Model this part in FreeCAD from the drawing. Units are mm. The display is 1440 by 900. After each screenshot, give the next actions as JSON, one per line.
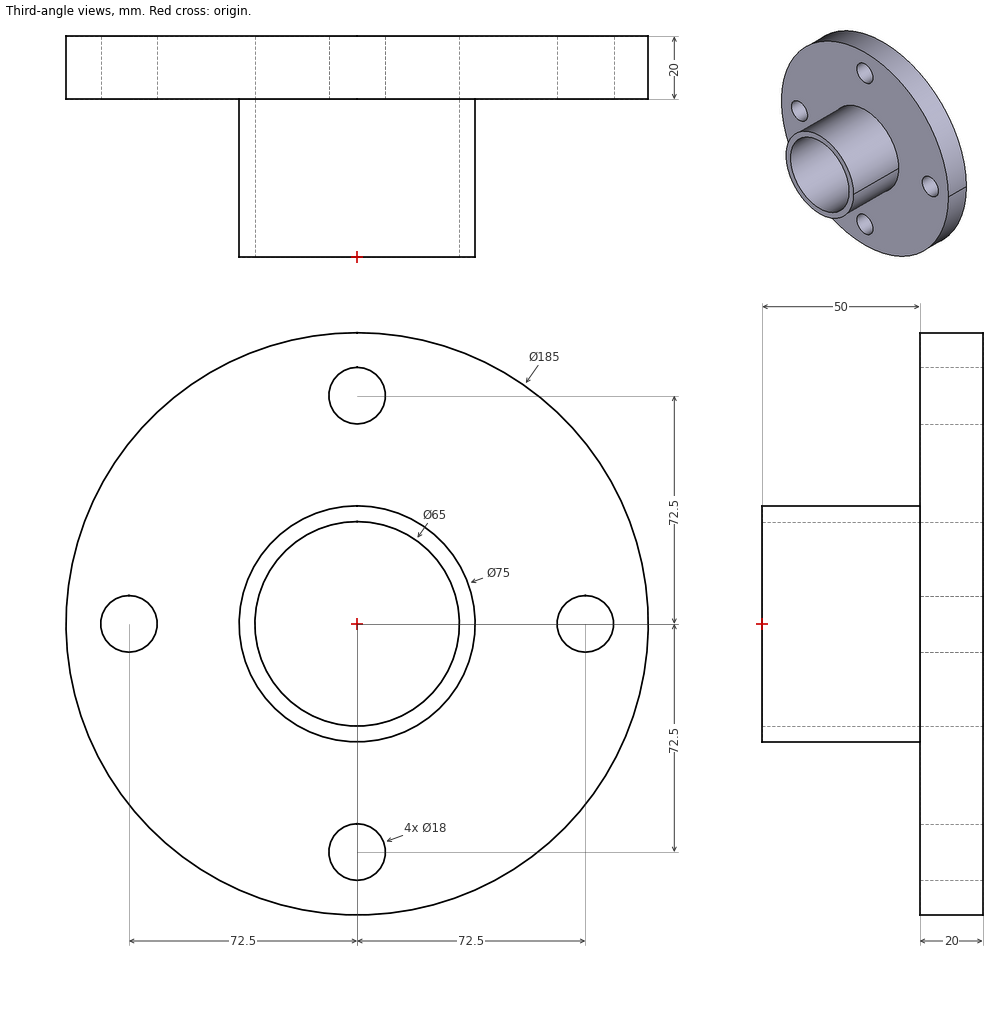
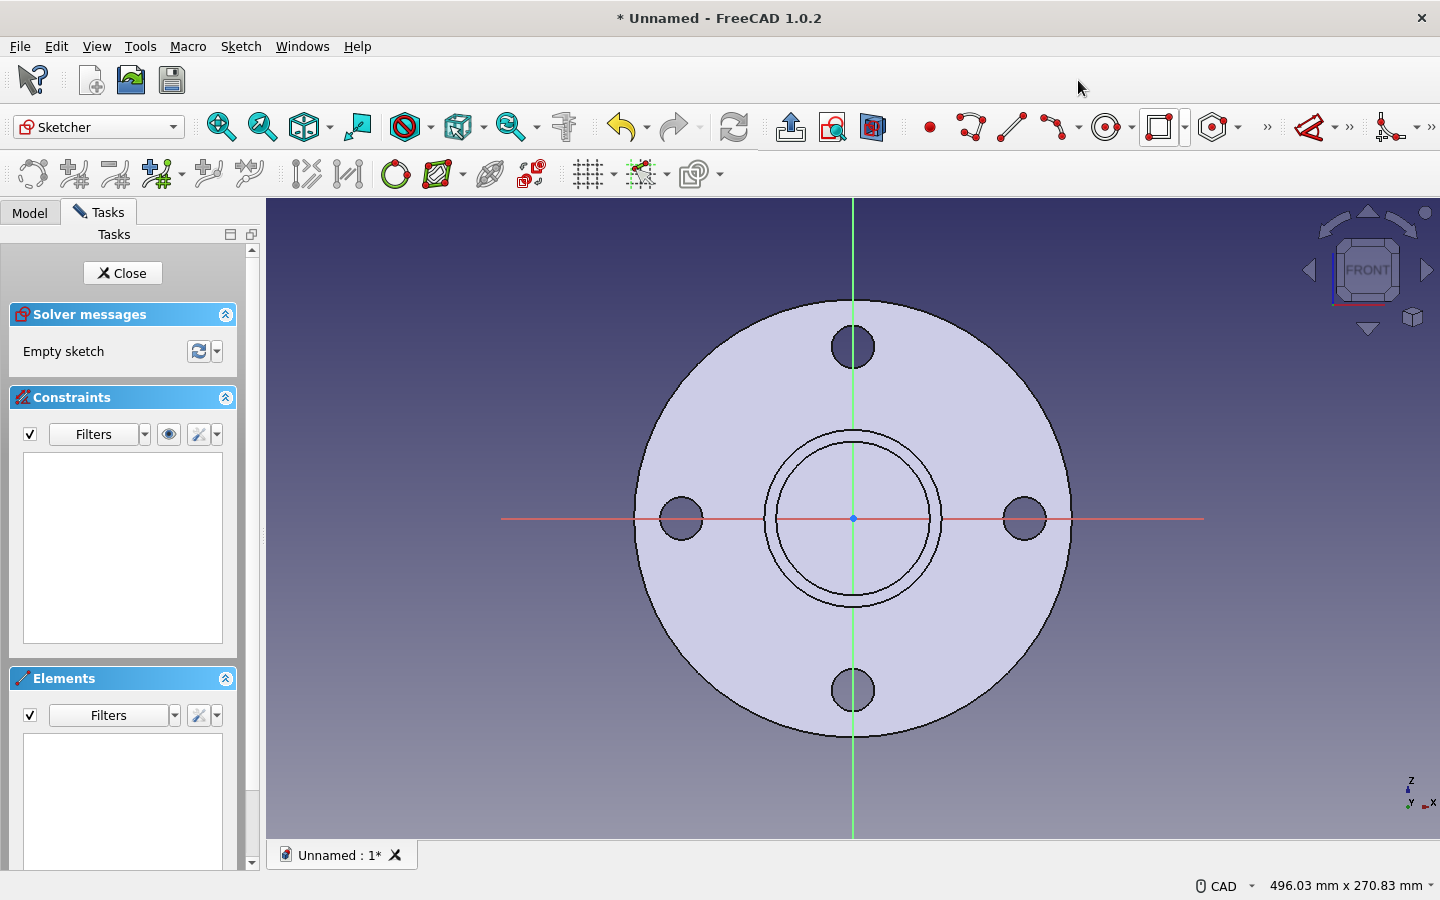
{"action": "scroll", "coordinate": [893, 518], "scroll_direction": "up", "scroll_amount": 5}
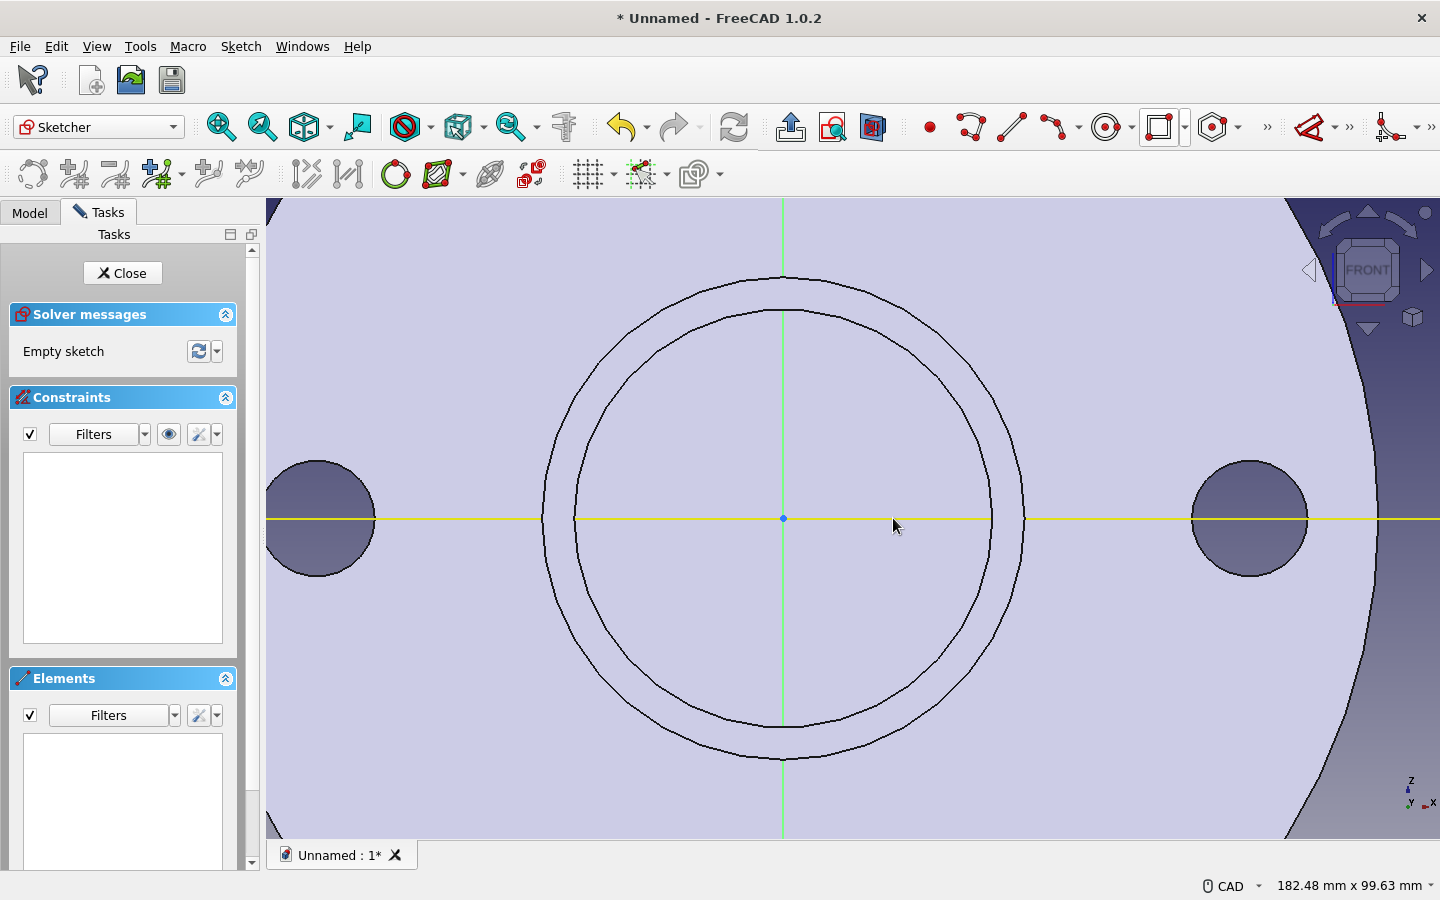
{"action": "key", "text": "g c"}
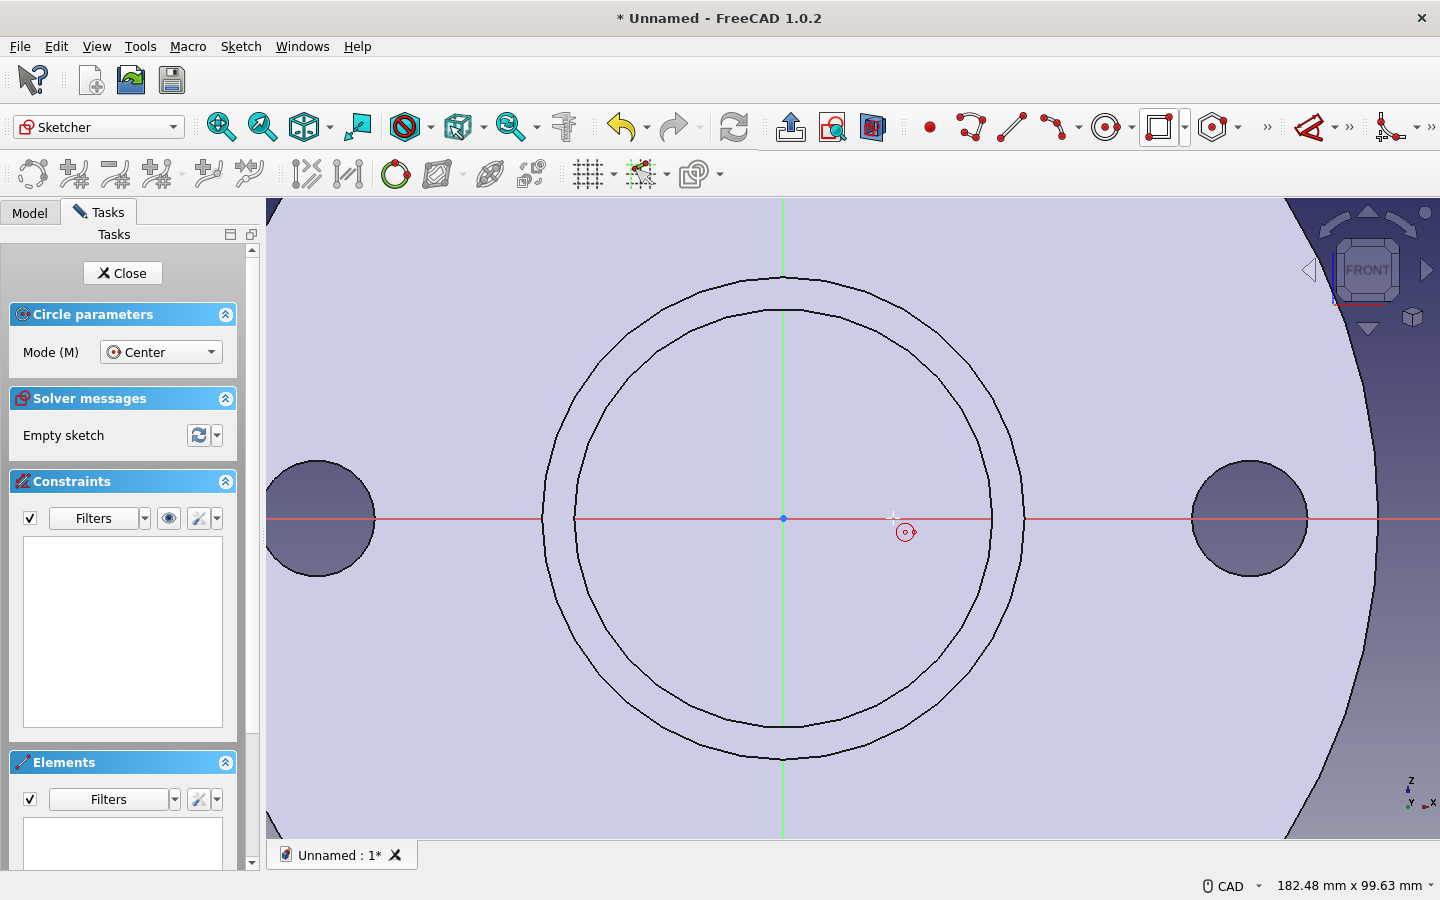
{"action": "left_click", "coordinate": [783, 518]}
{"action": "left_click", "coordinate": [931, 371]}
{"action": "key", "text": "Escape"}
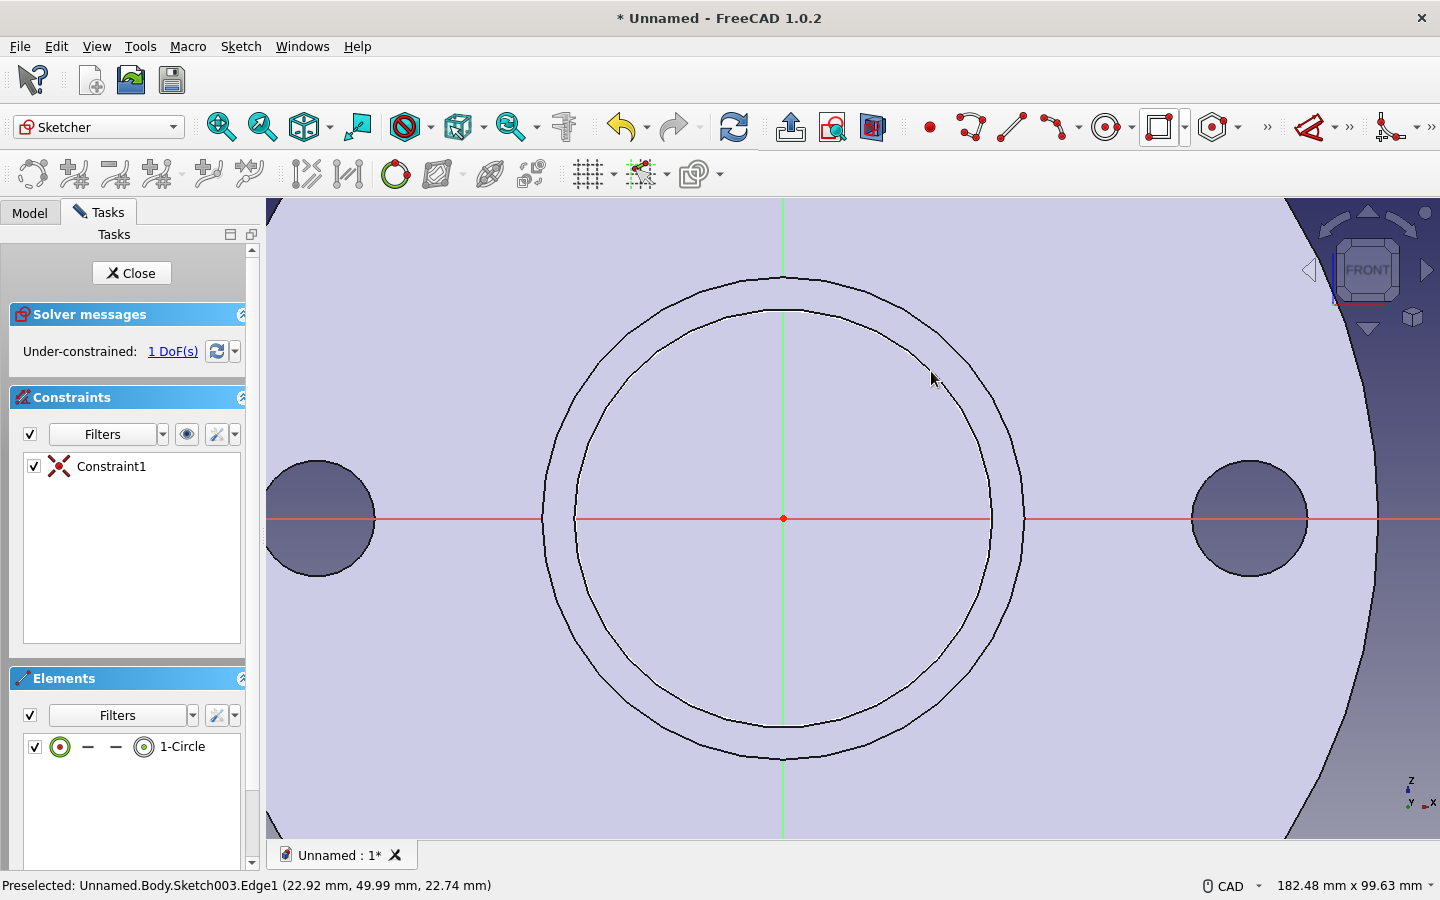
{"action": "left_click", "coordinate": [1308, 128]}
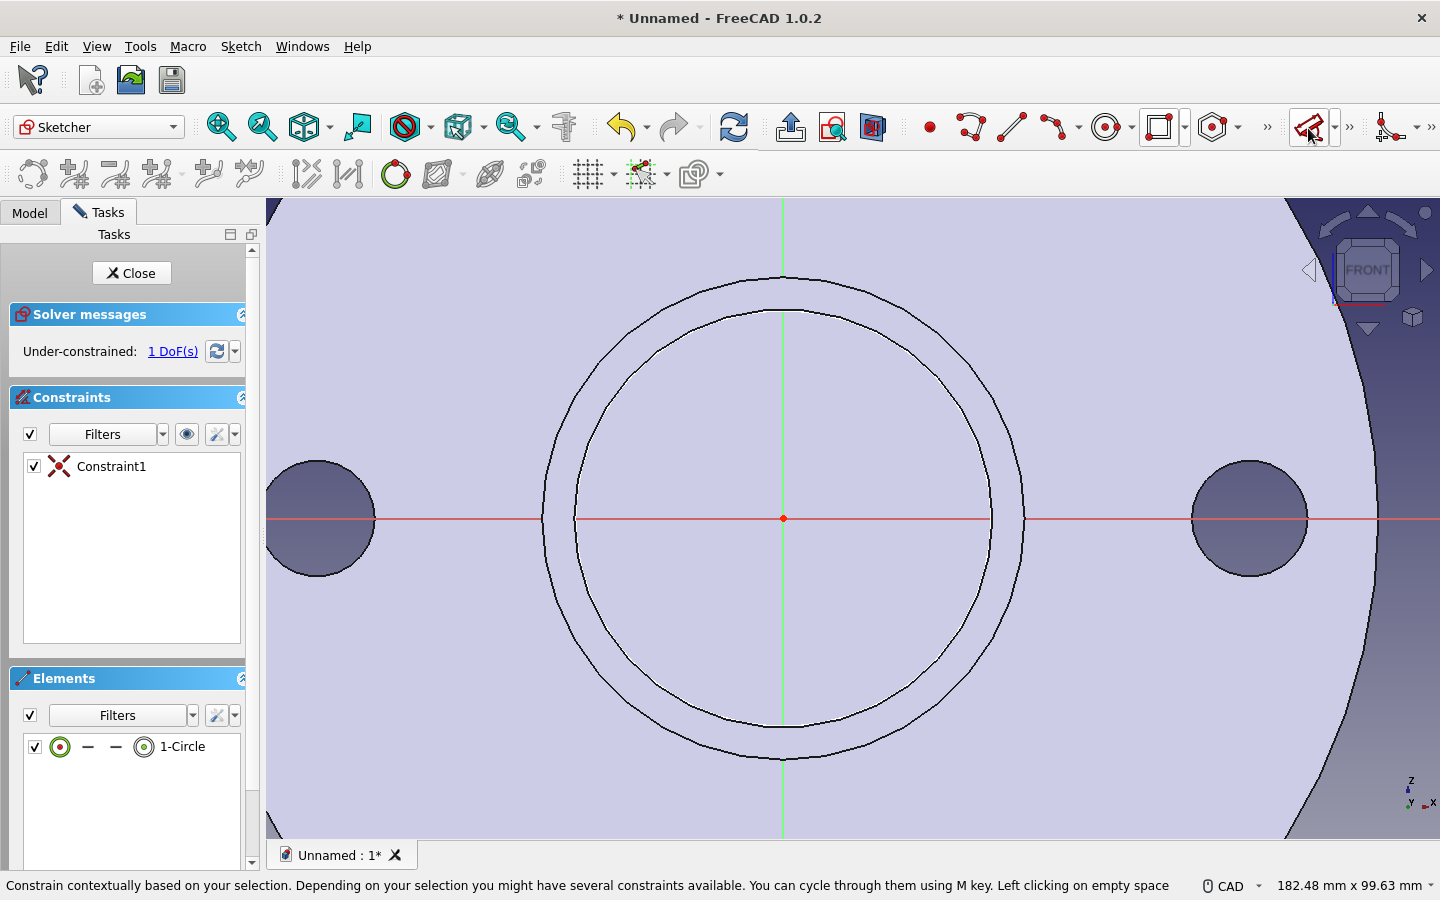
{"action": "left_click", "coordinate": [930, 371]}
{"action": "left_click", "coordinate": [953, 348]}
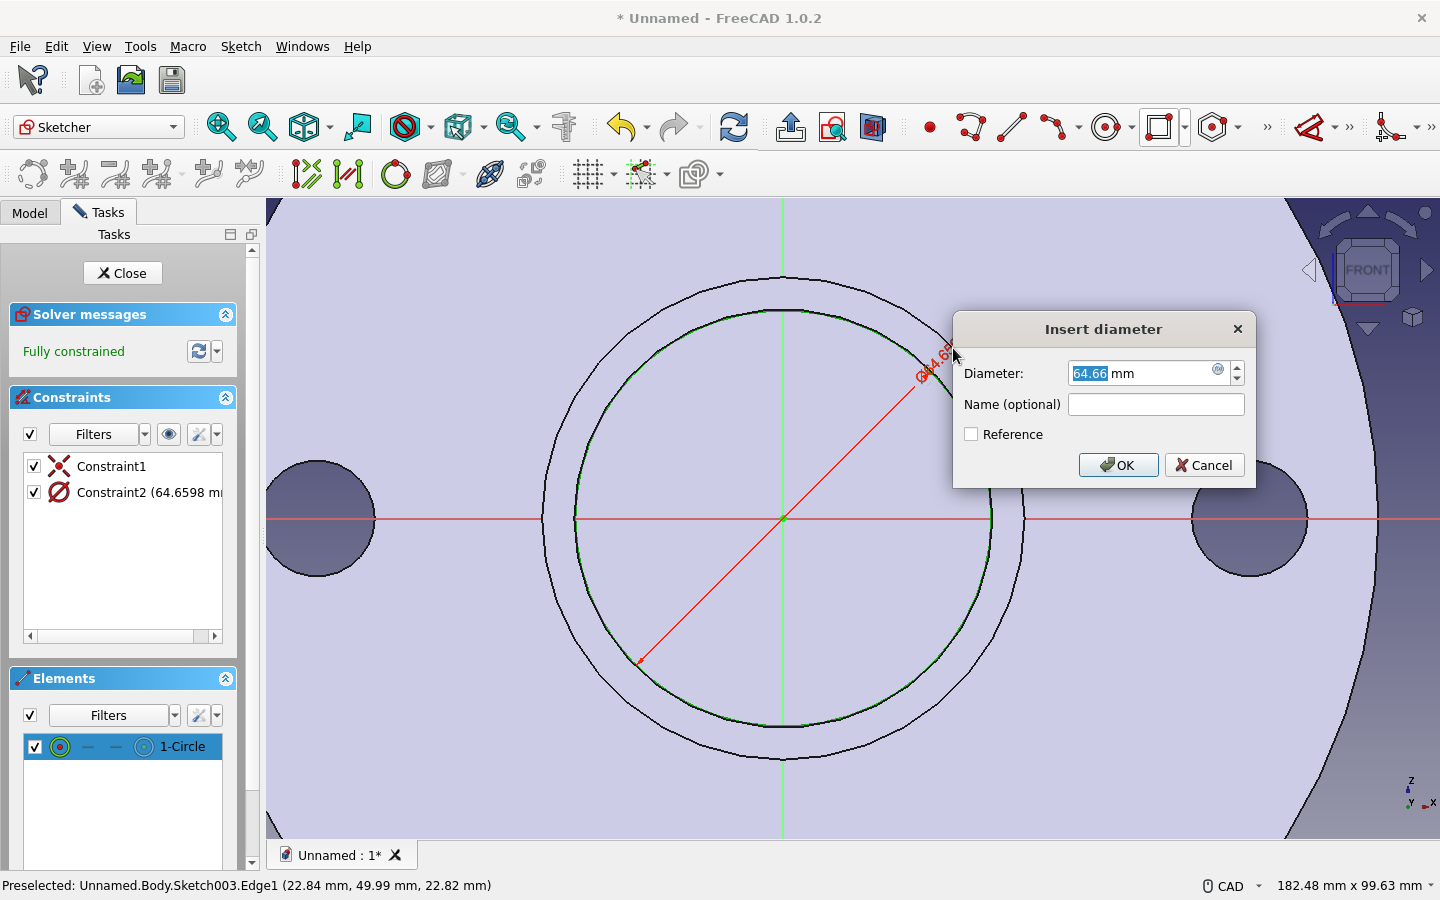
{"action": "type", "text": "65"}
{"action": "key", "text": "Return"}
{"action": "key", "text": "Escape"}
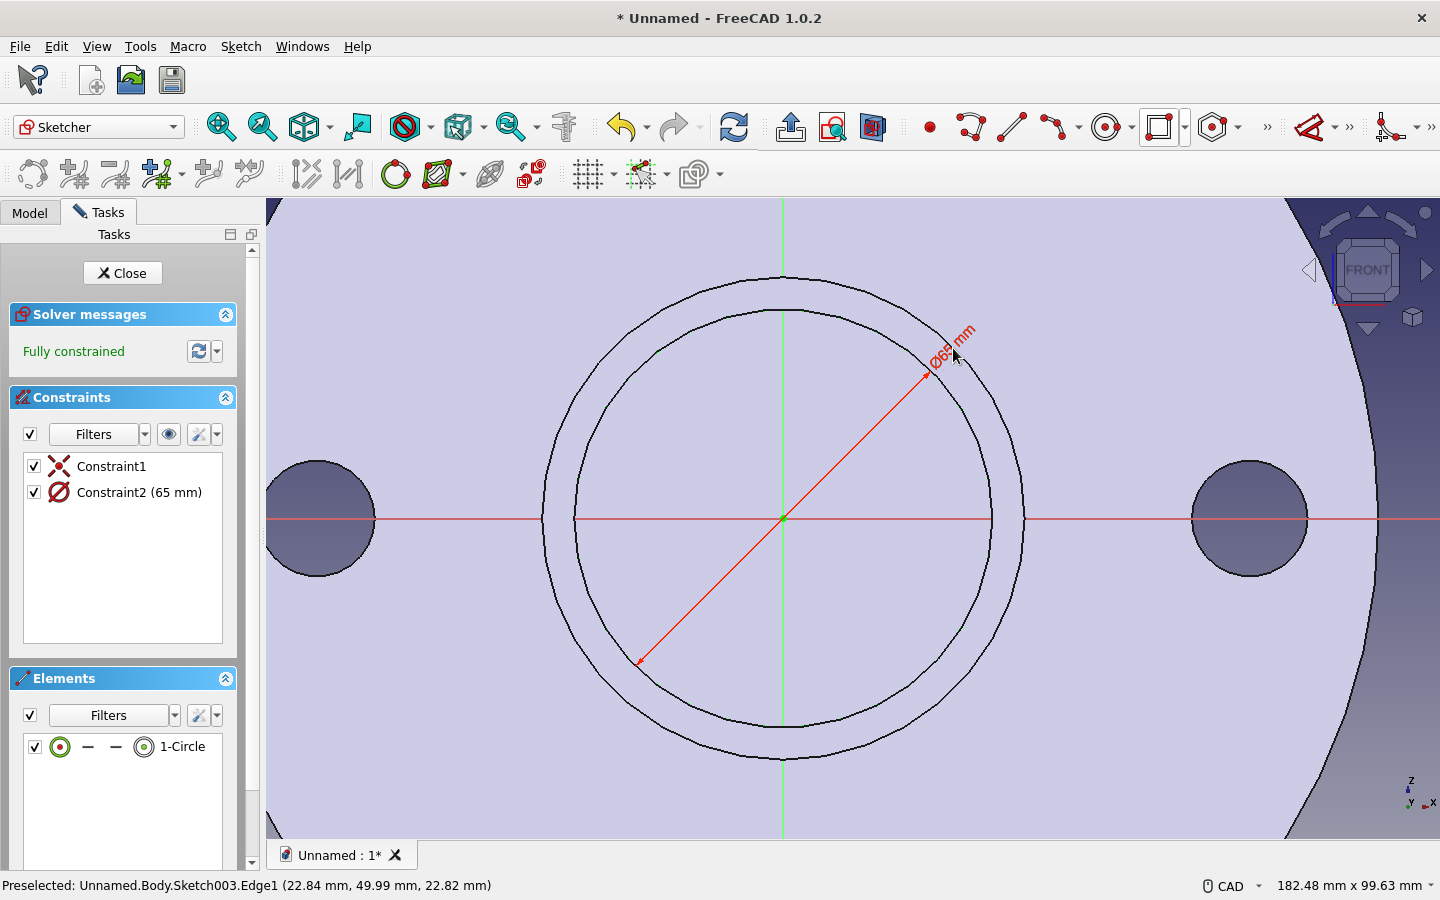
{"action": "left_click", "coordinate": [123, 273]}